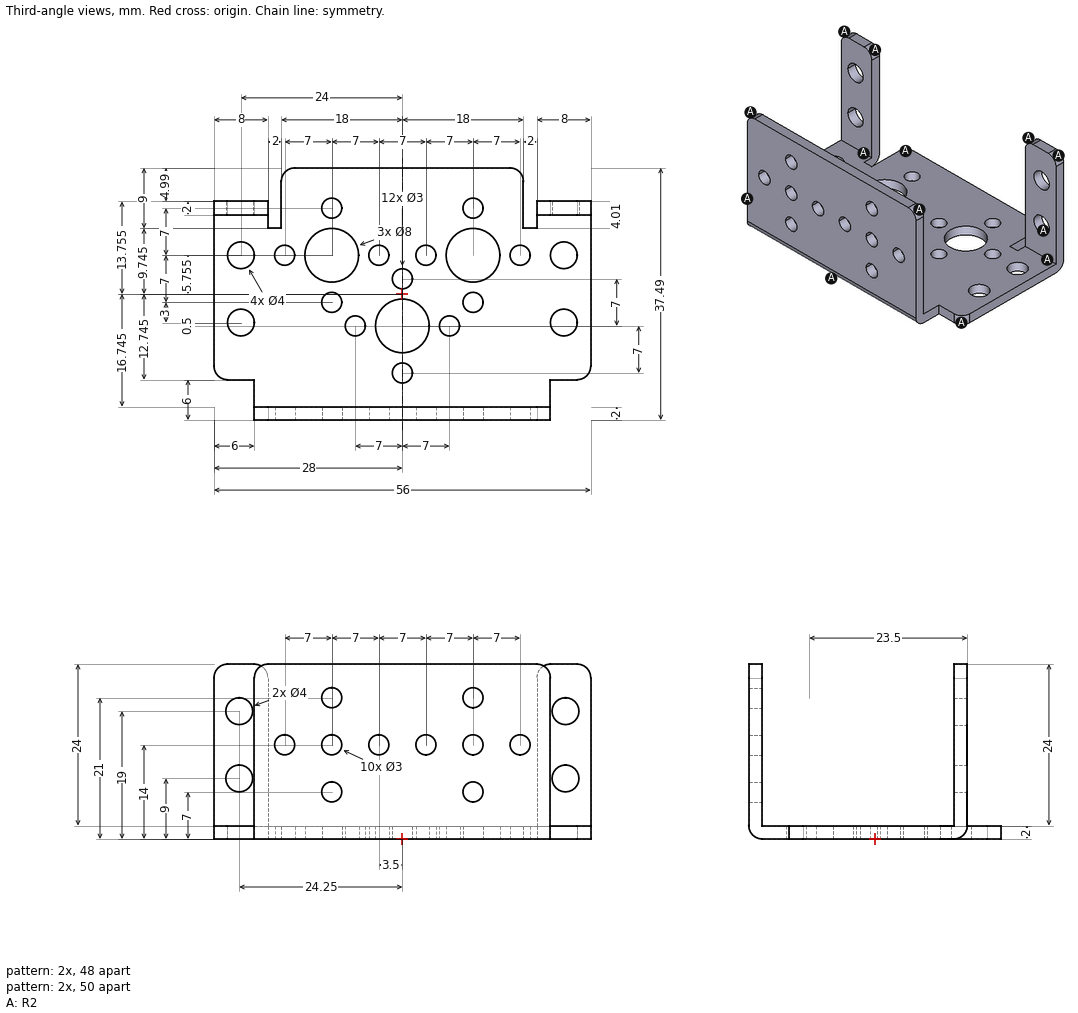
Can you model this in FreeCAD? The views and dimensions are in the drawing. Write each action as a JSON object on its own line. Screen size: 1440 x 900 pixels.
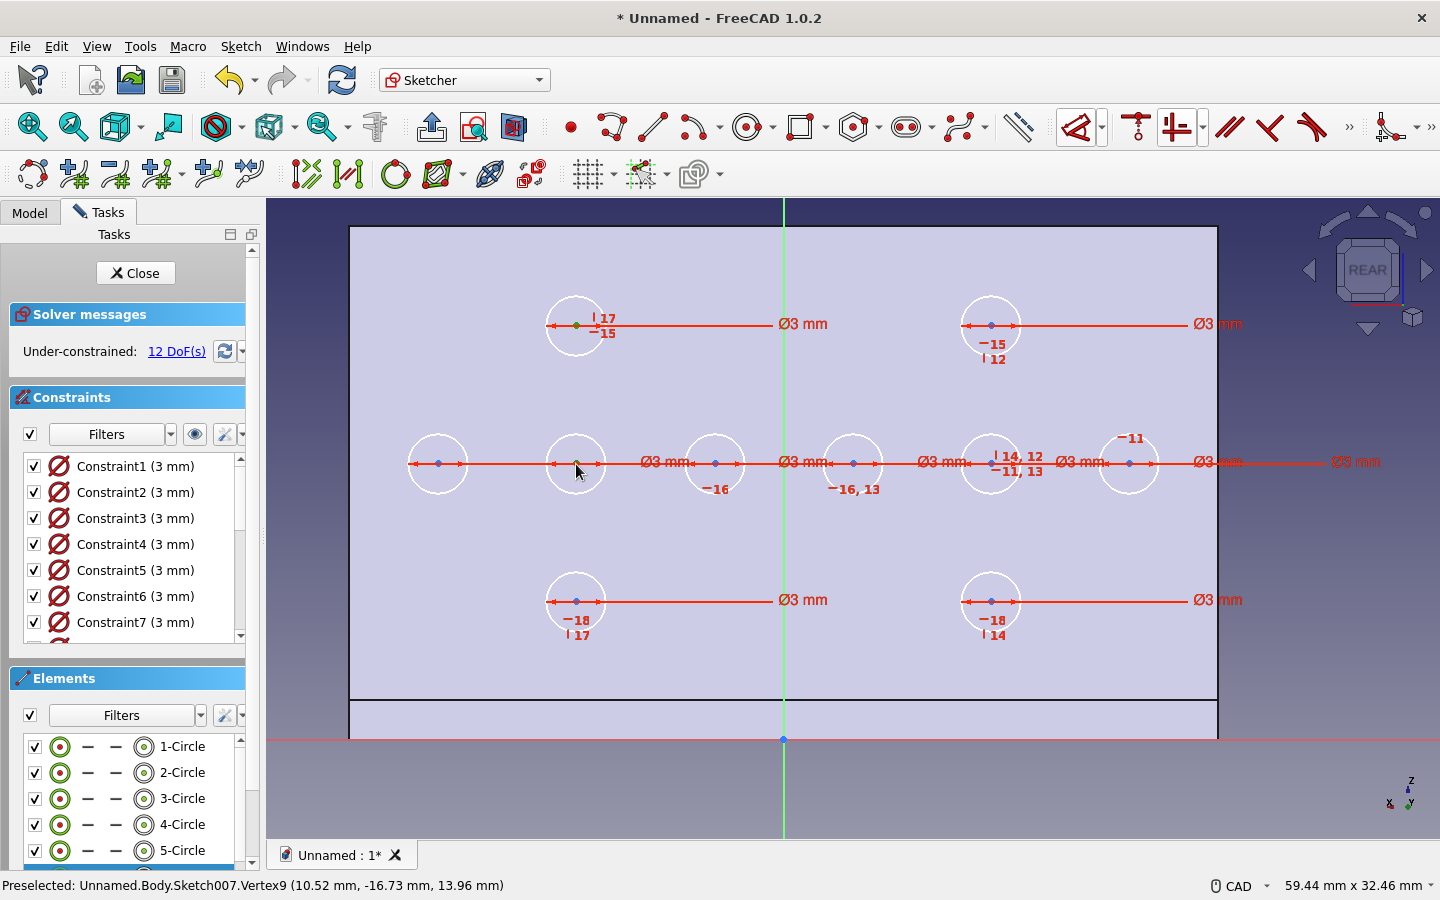
{"action": "key", "text": "v"}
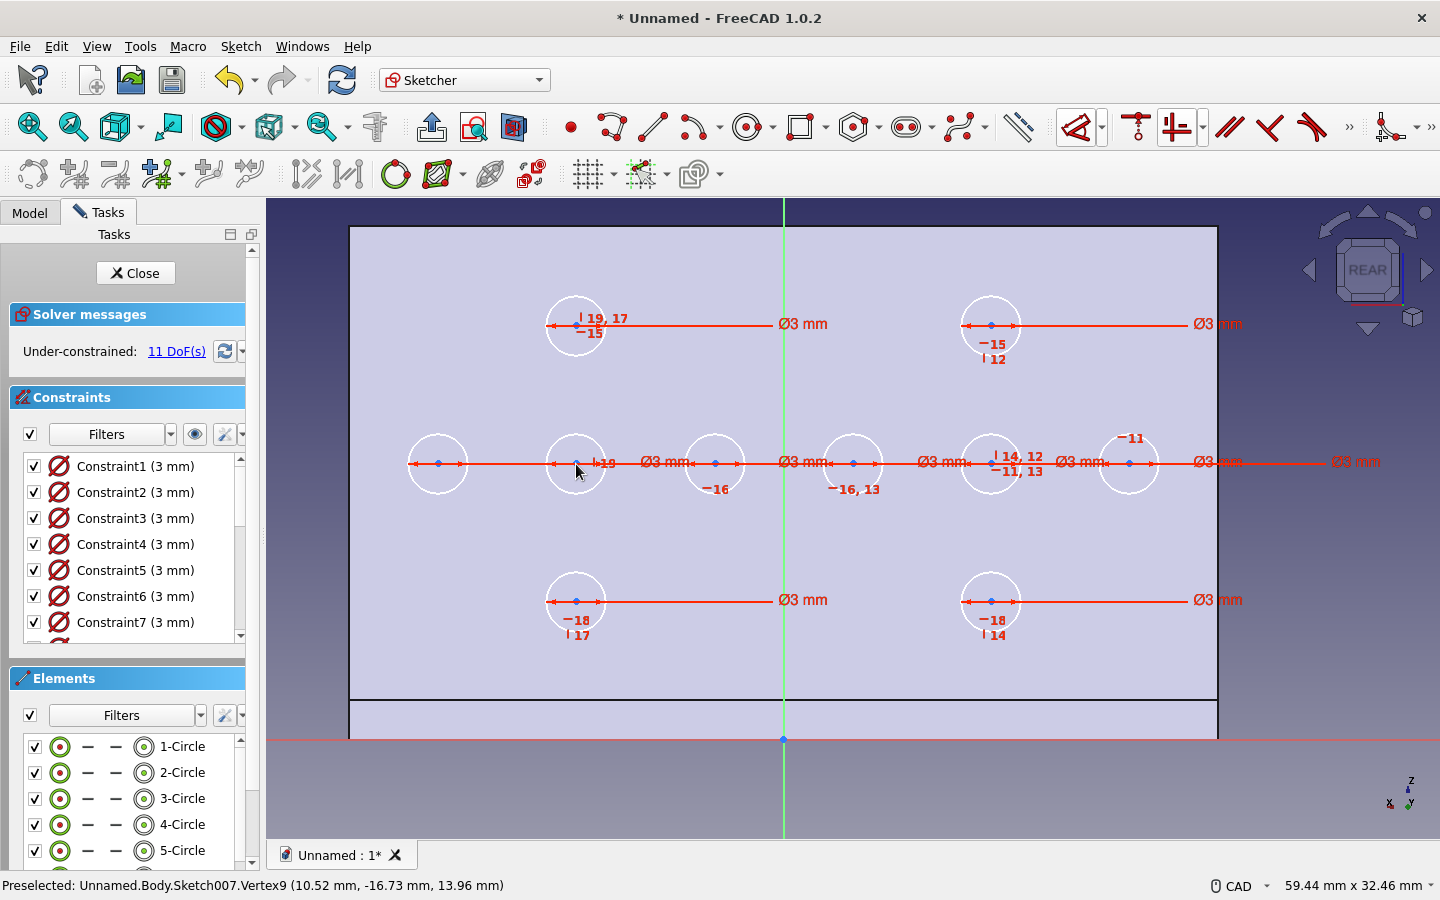
{"action": "left_click", "coordinate": [715, 464]}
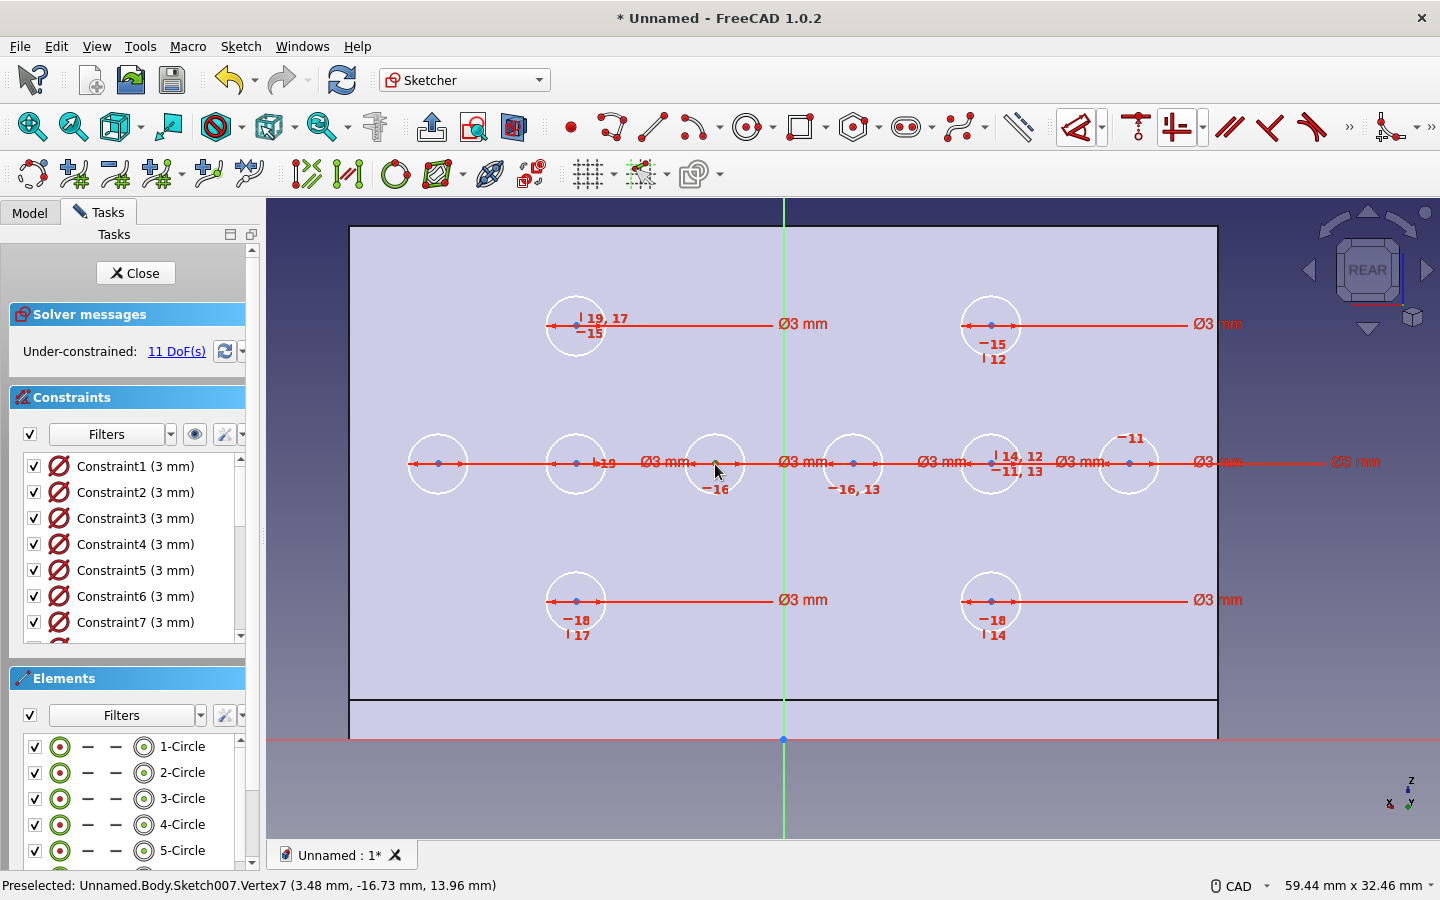
{"action": "left_click", "coordinate": [576, 464]}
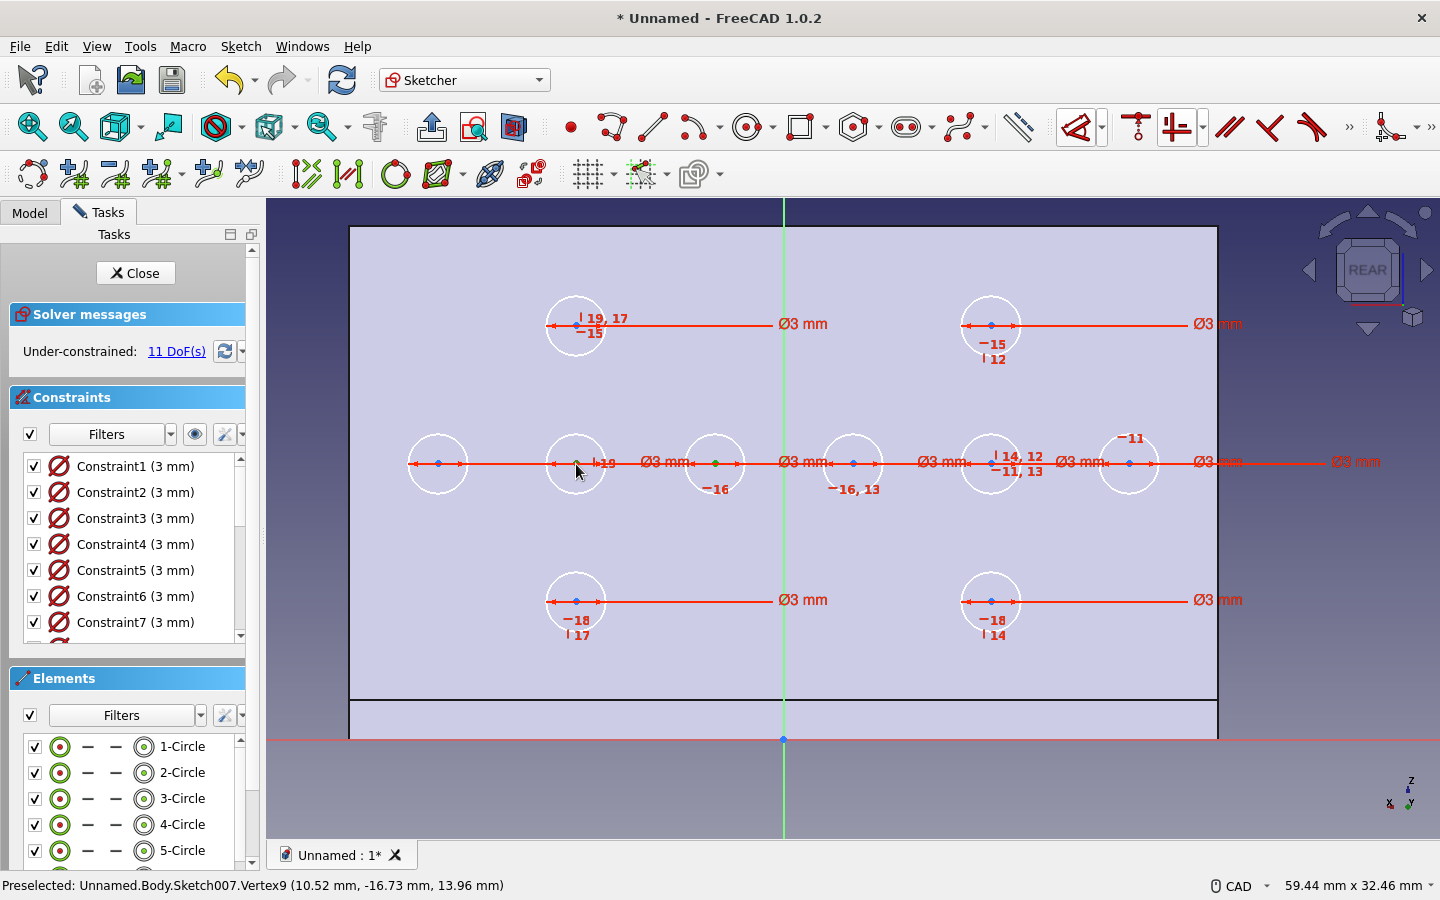
{"action": "key", "text": "h"}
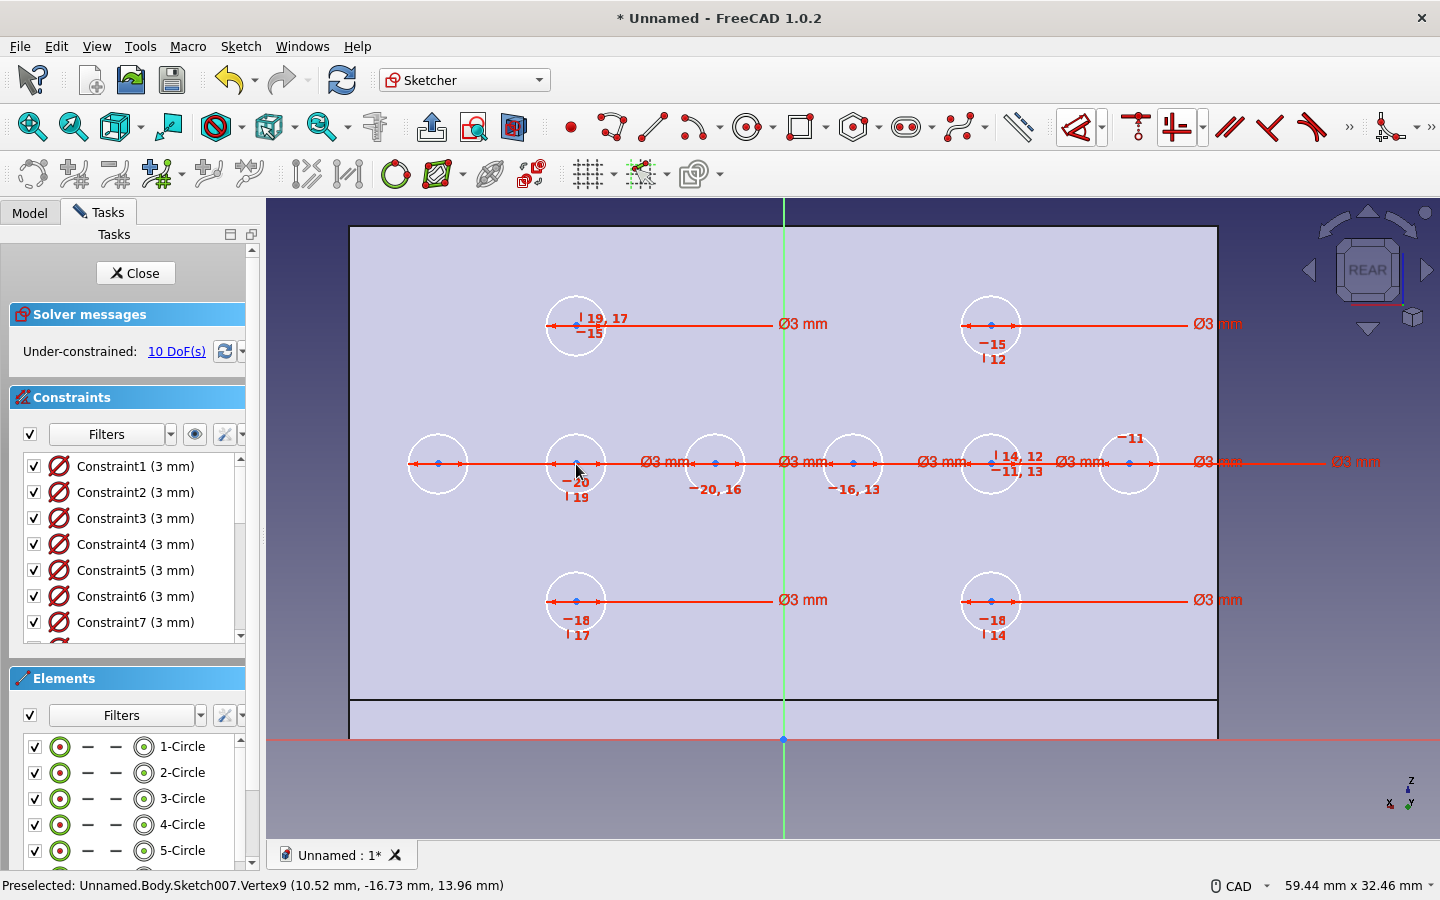
{"action": "left_click", "coordinate": [576, 464]}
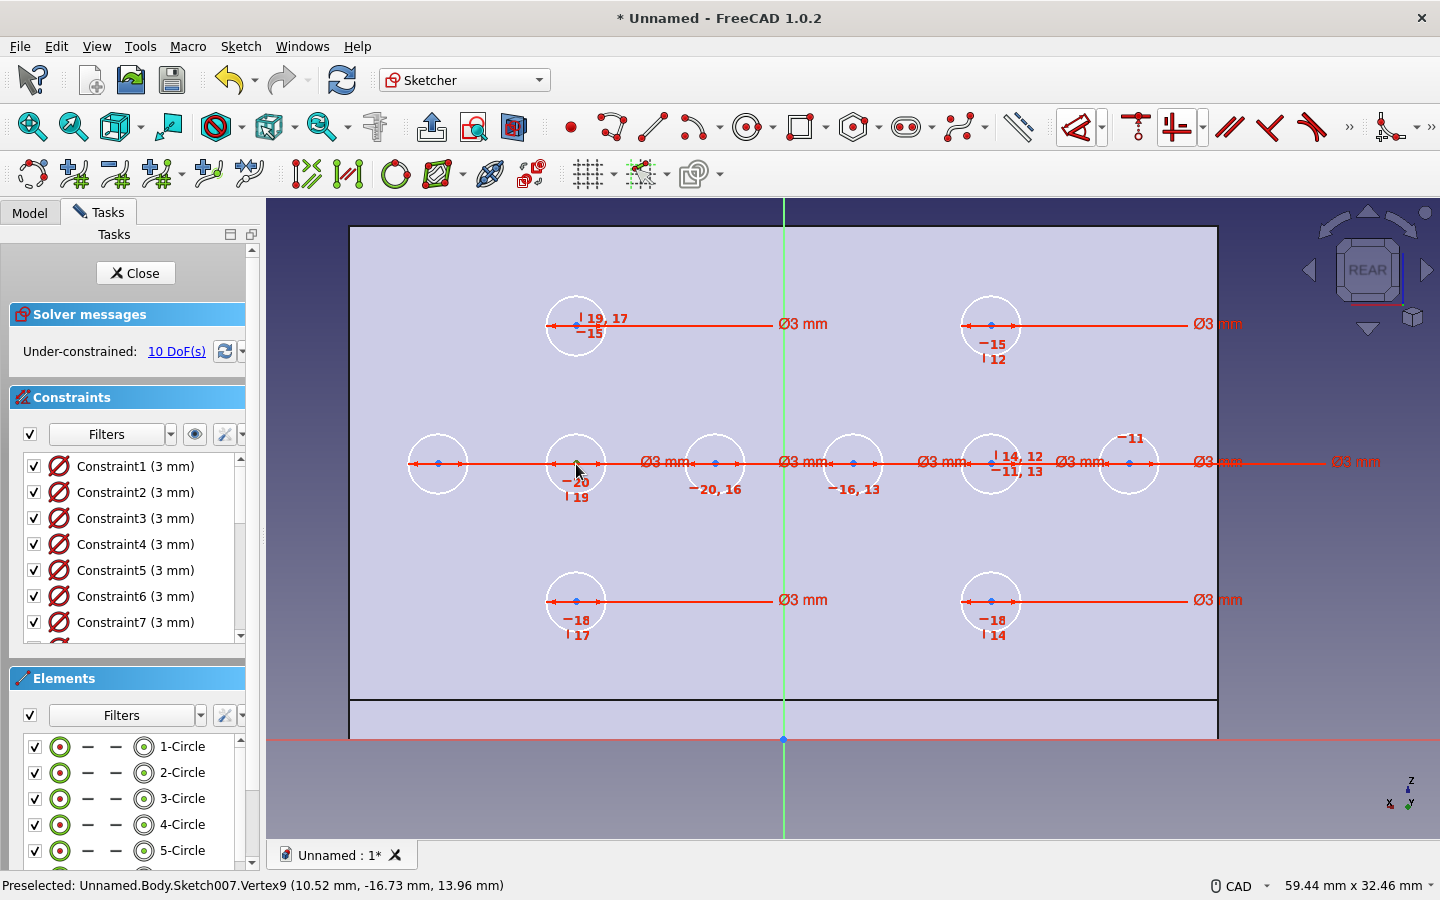
{"action": "left_click", "coordinate": [438, 464]}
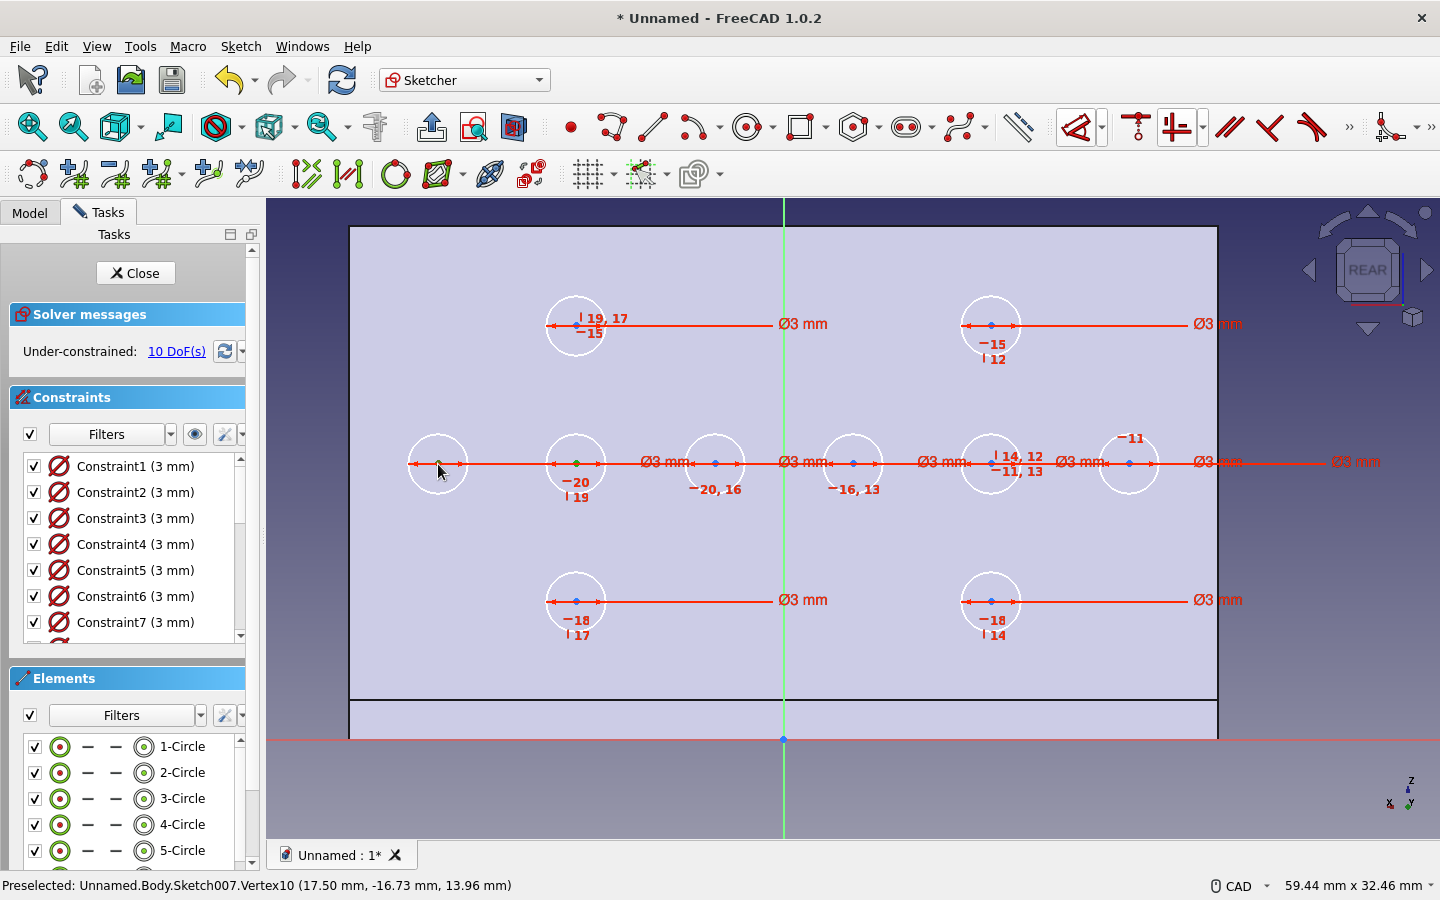
{"action": "key", "text": "h"}